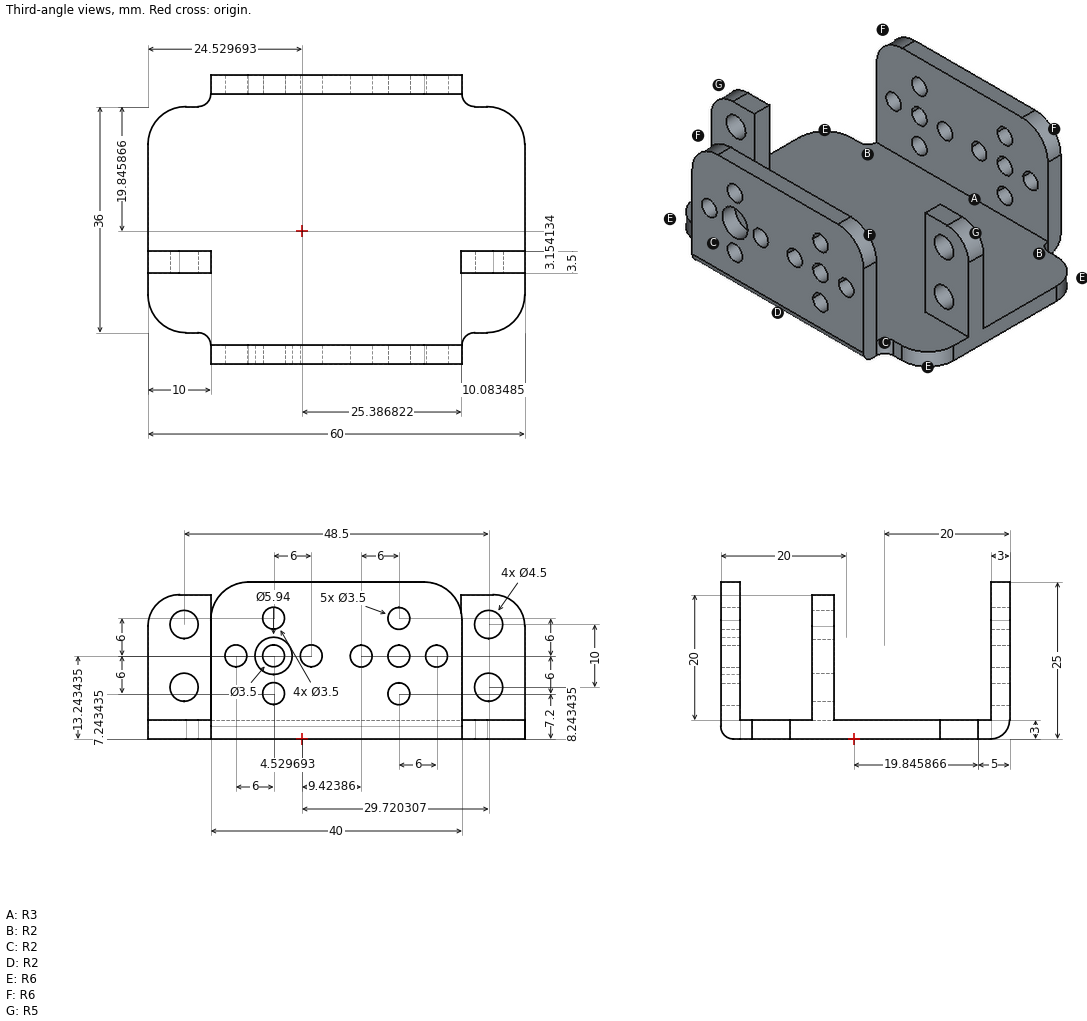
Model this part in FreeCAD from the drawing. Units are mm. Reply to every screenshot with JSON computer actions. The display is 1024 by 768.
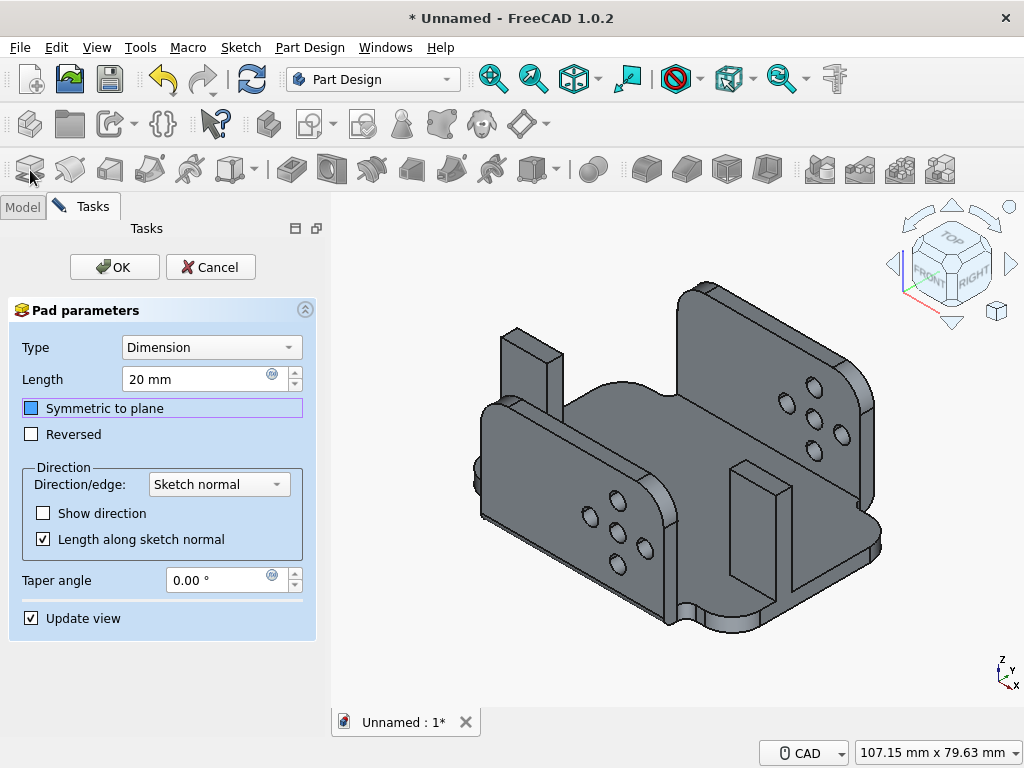
{"action": "left_click", "coordinate": [115, 267]}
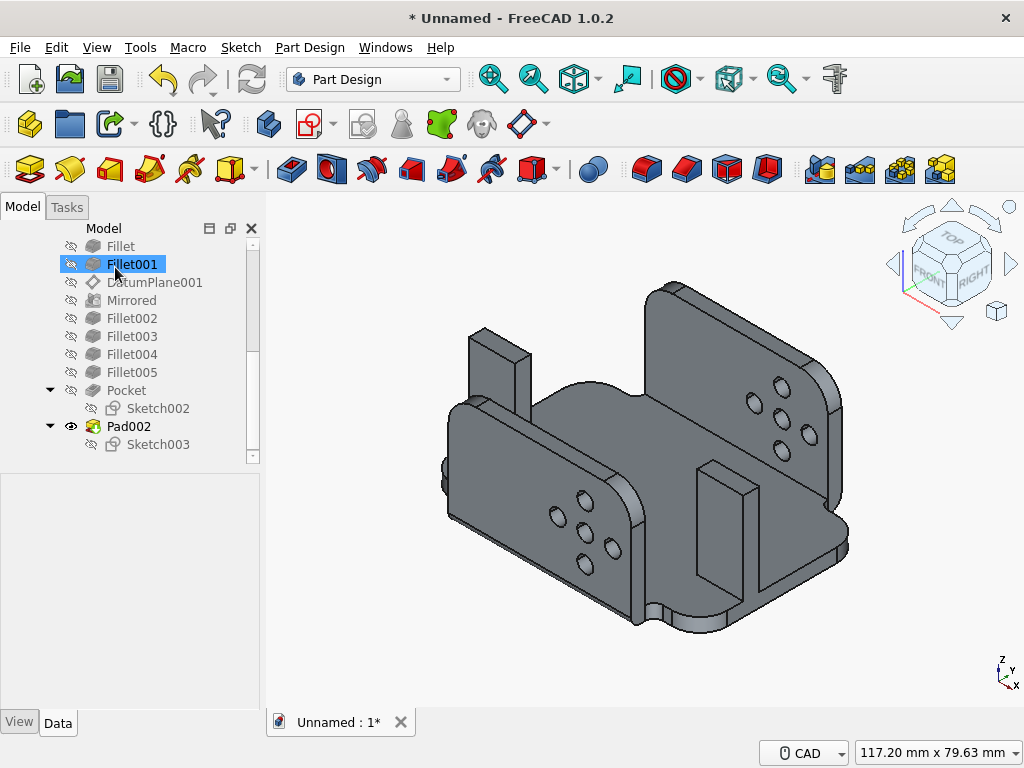
{"action": "left_click", "coordinate": [751, 490]}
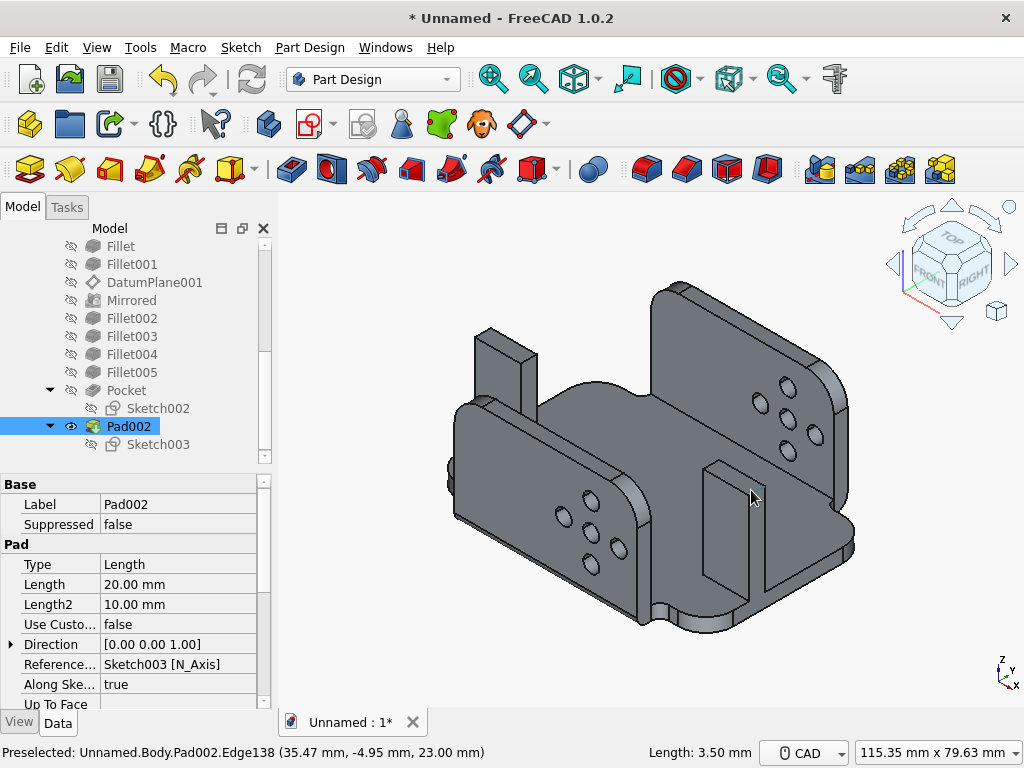
{"action": "key", "text": "2"}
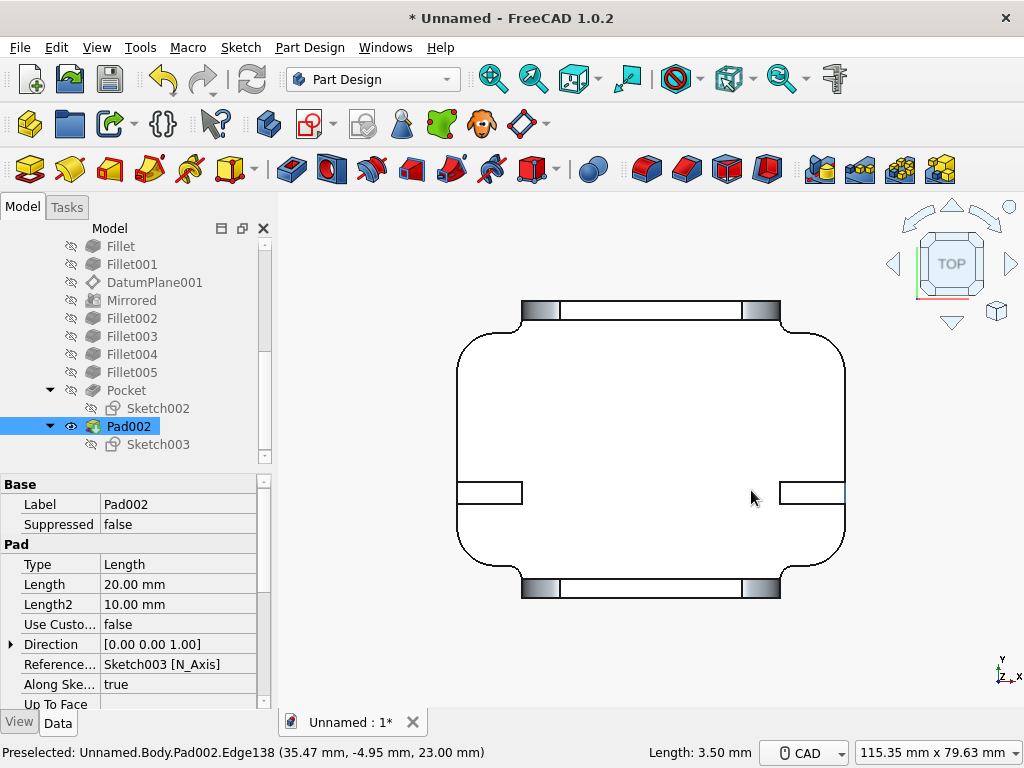
{"action": "left_click", "coordinate": [457, 492], "text": "ctrl"}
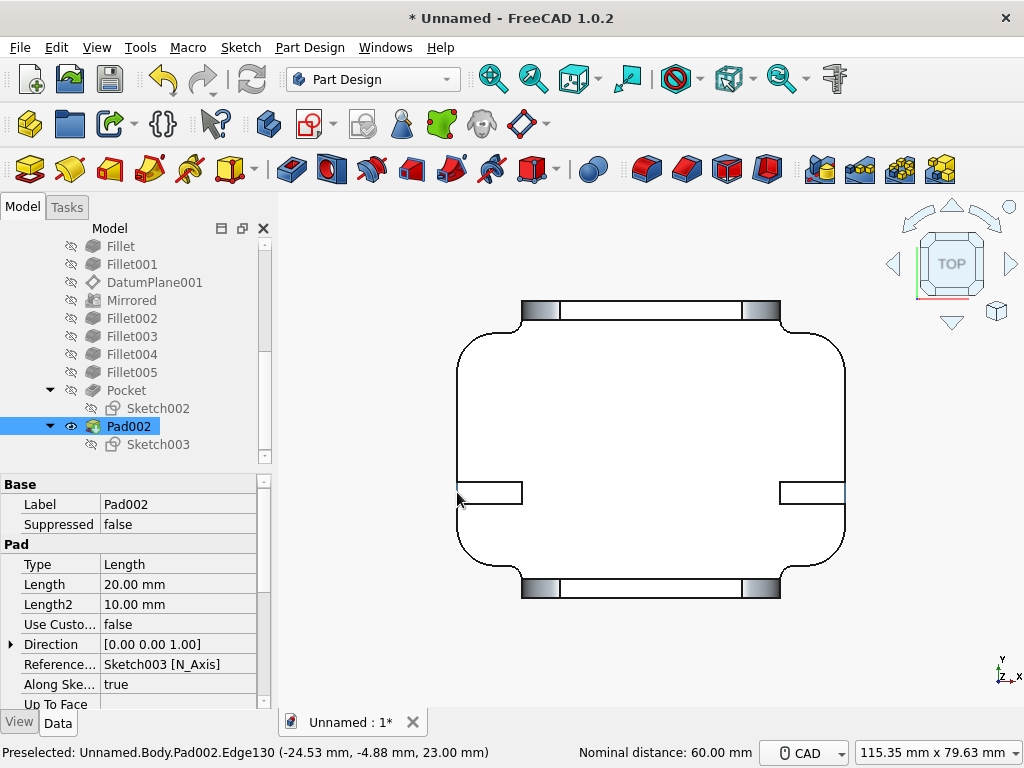
{"action": "left_click", "coordinate": [648, 170]}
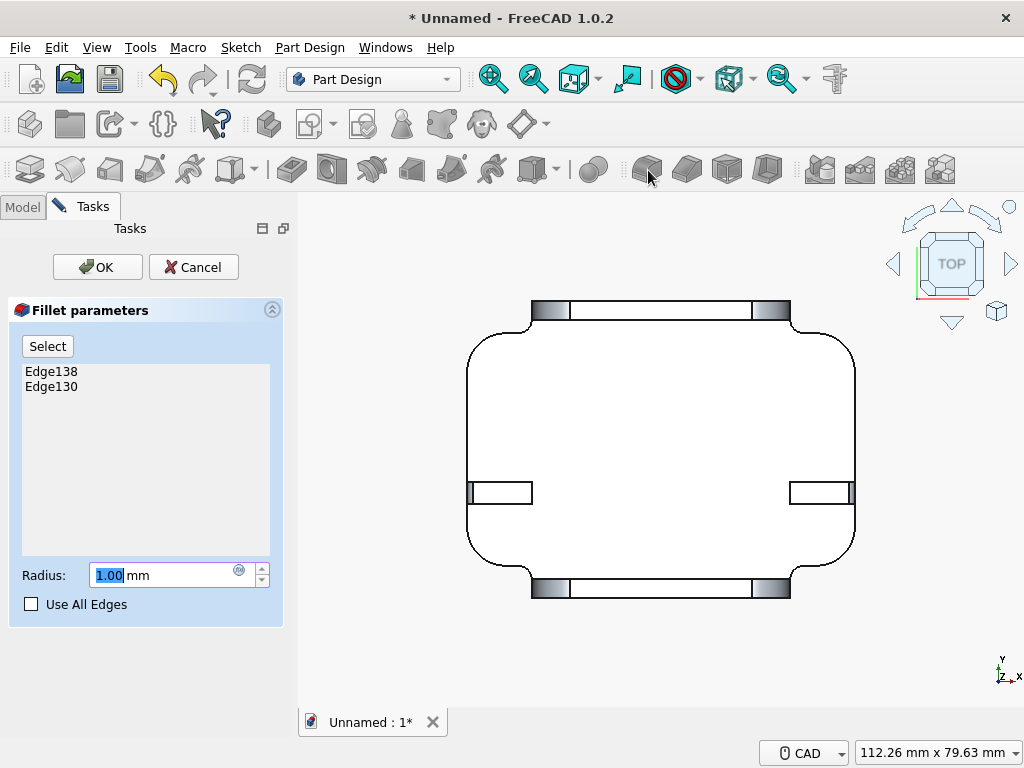
{"action": "type", "text": "5"}
{"action": "key", "text": "Tab"}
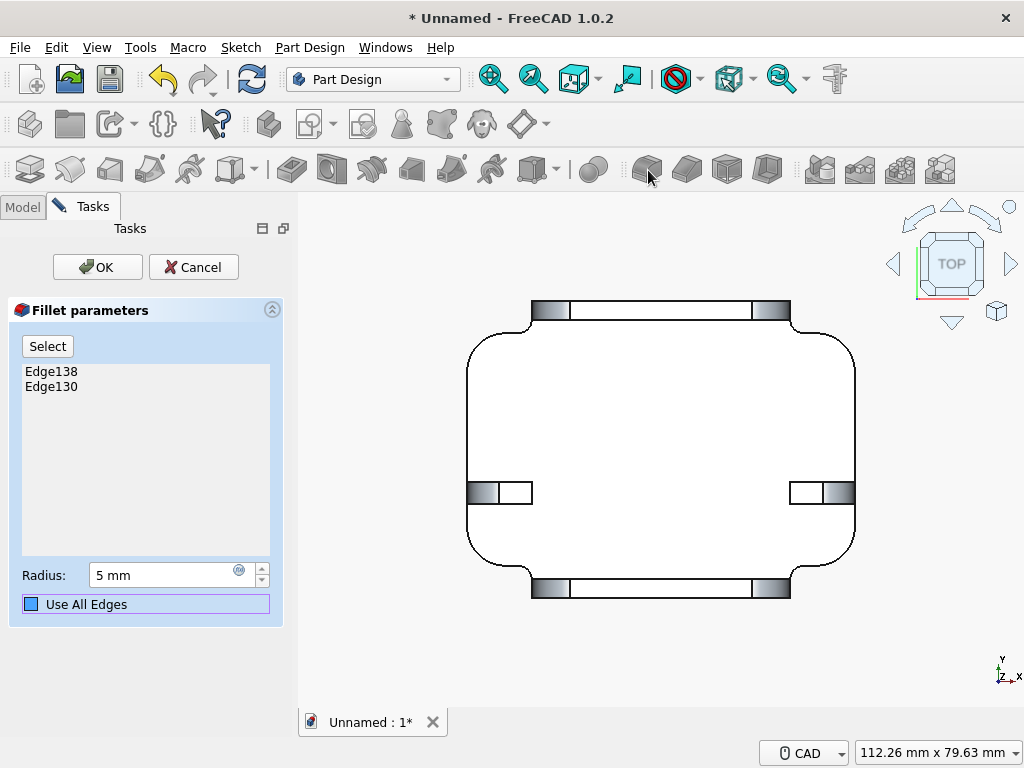
{"action": "left_click", "coordinate": [98, 267]}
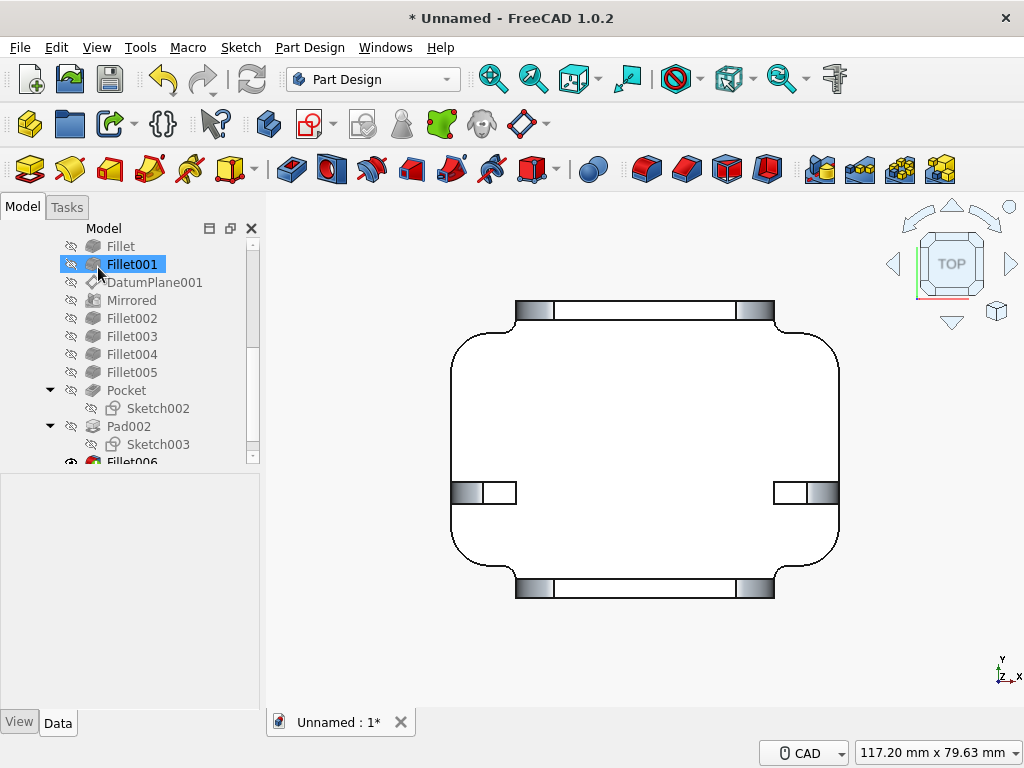
{"action": "key", "text": "0"}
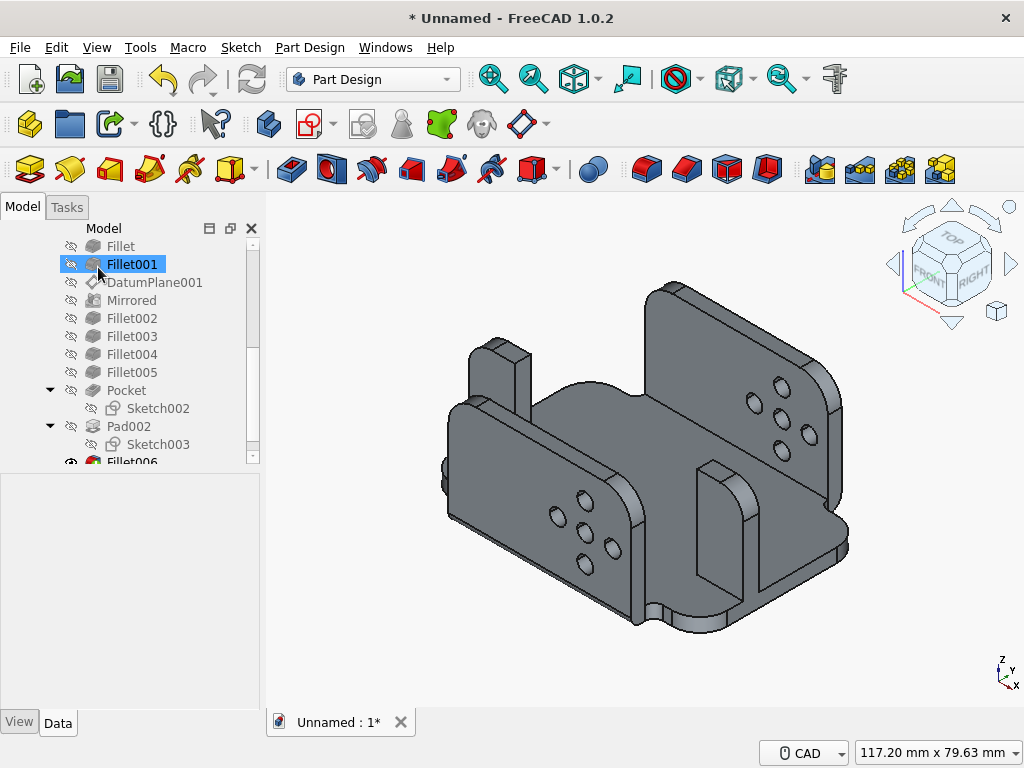
{"action": "left_click", "coordinate": [720, 519]}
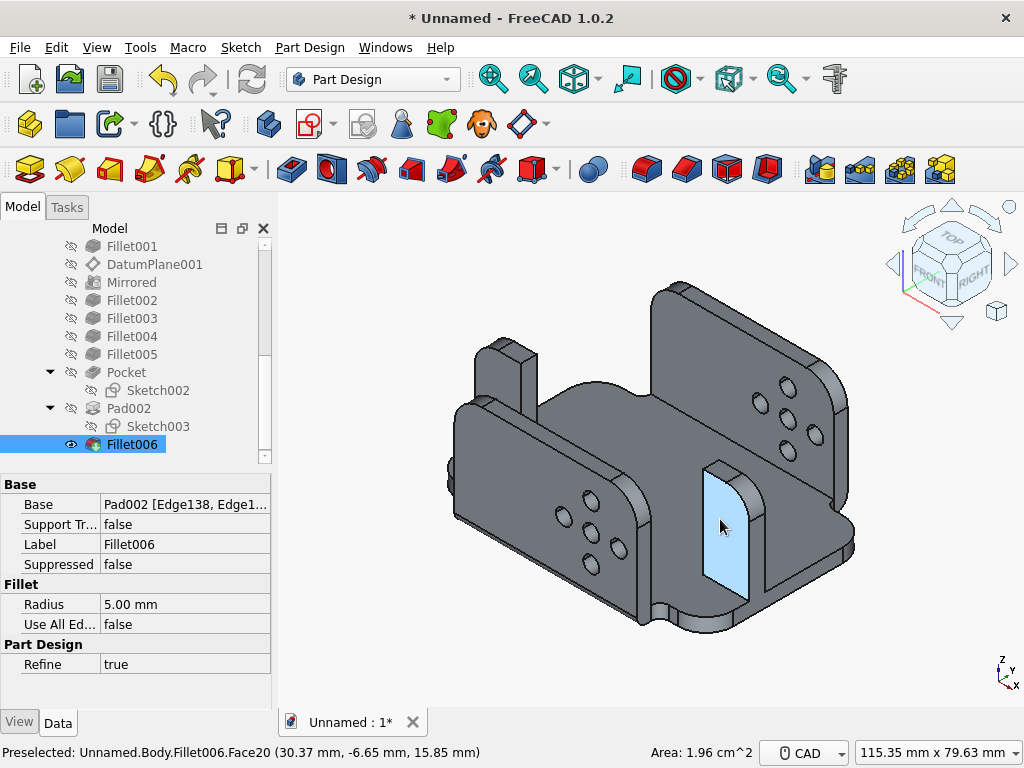
{"action": "left_click", "coordinate": [310, 124]}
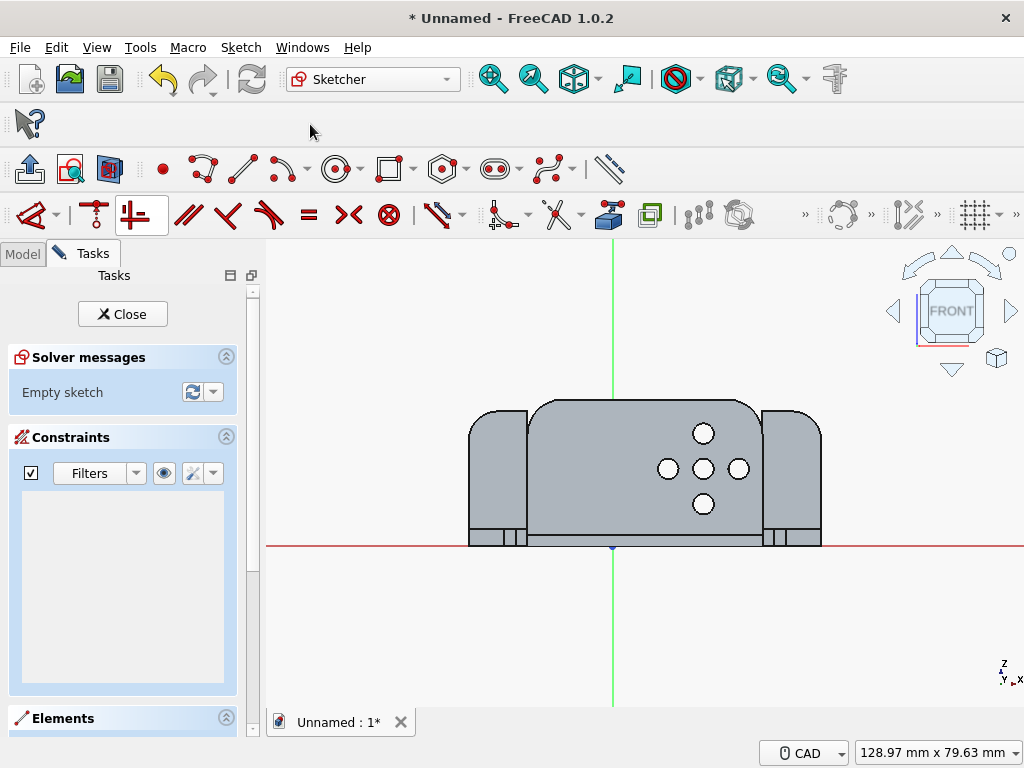
{"action": "left_click", "coordinate": [336, 170]}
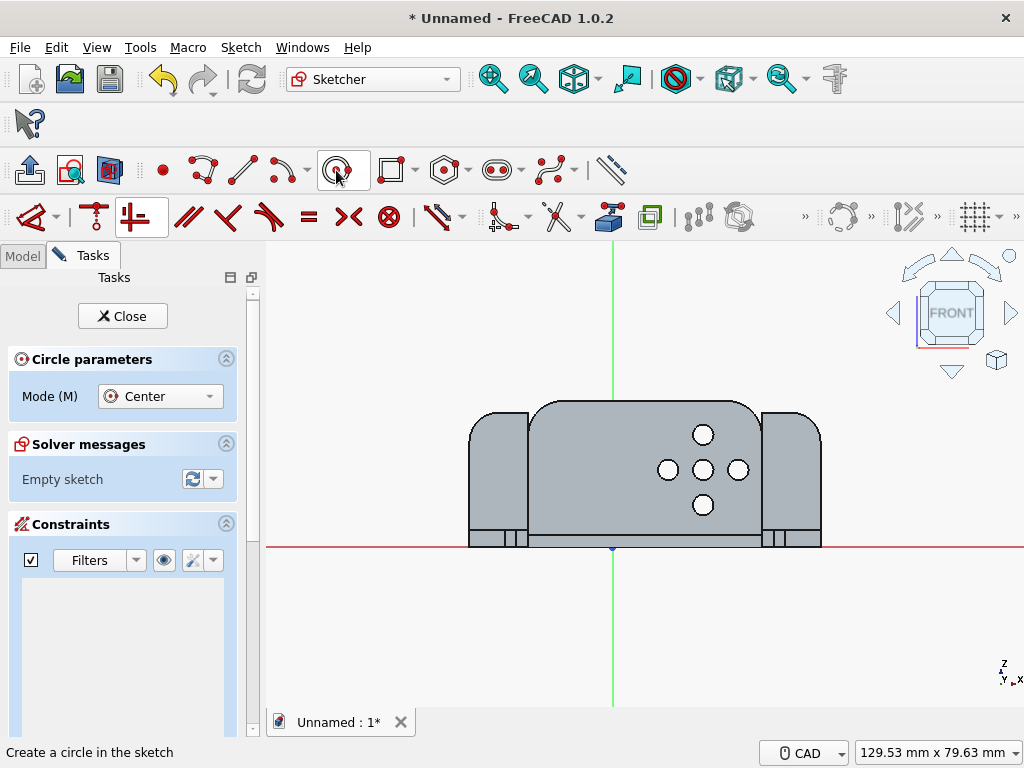
{"action": "scroll", "coordinate": [787, 440], "scroll_direction": "up", "scroll_amount": 3}